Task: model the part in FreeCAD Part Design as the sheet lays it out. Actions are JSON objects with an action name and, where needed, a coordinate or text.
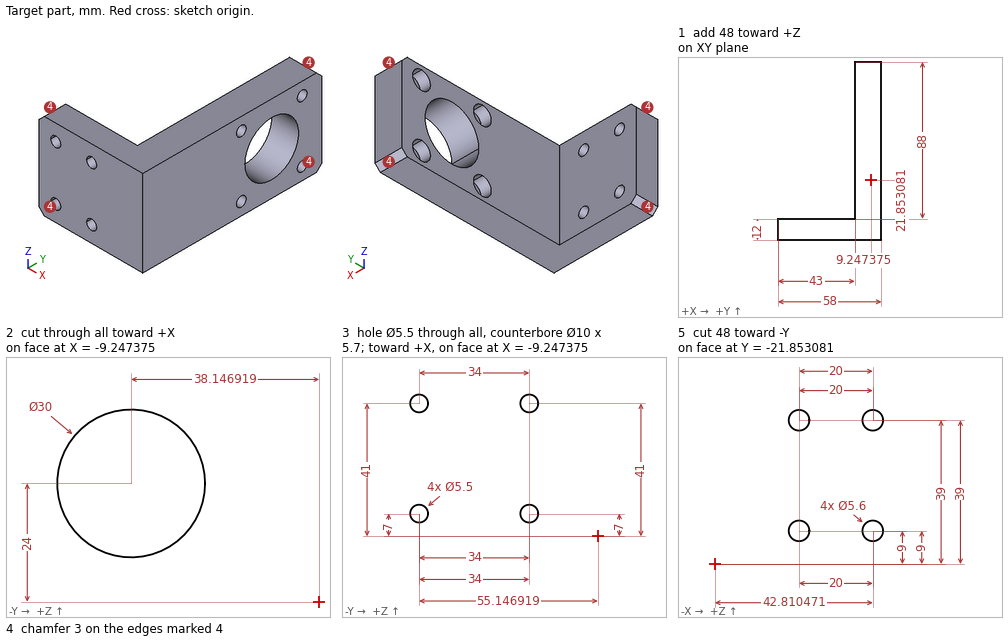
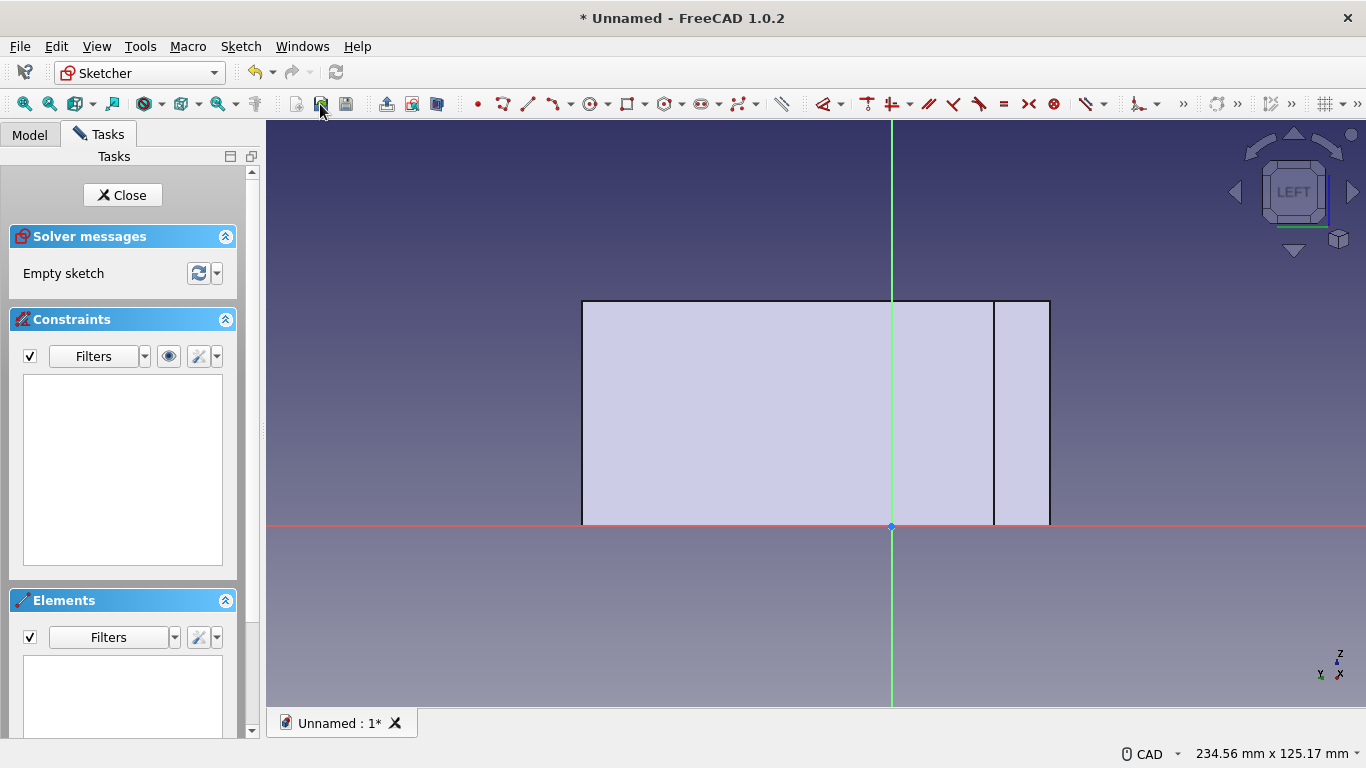
{"action": "scroll", "coordinate": [783, 452], "scroll_direction": "up", "scroll_amount": 4}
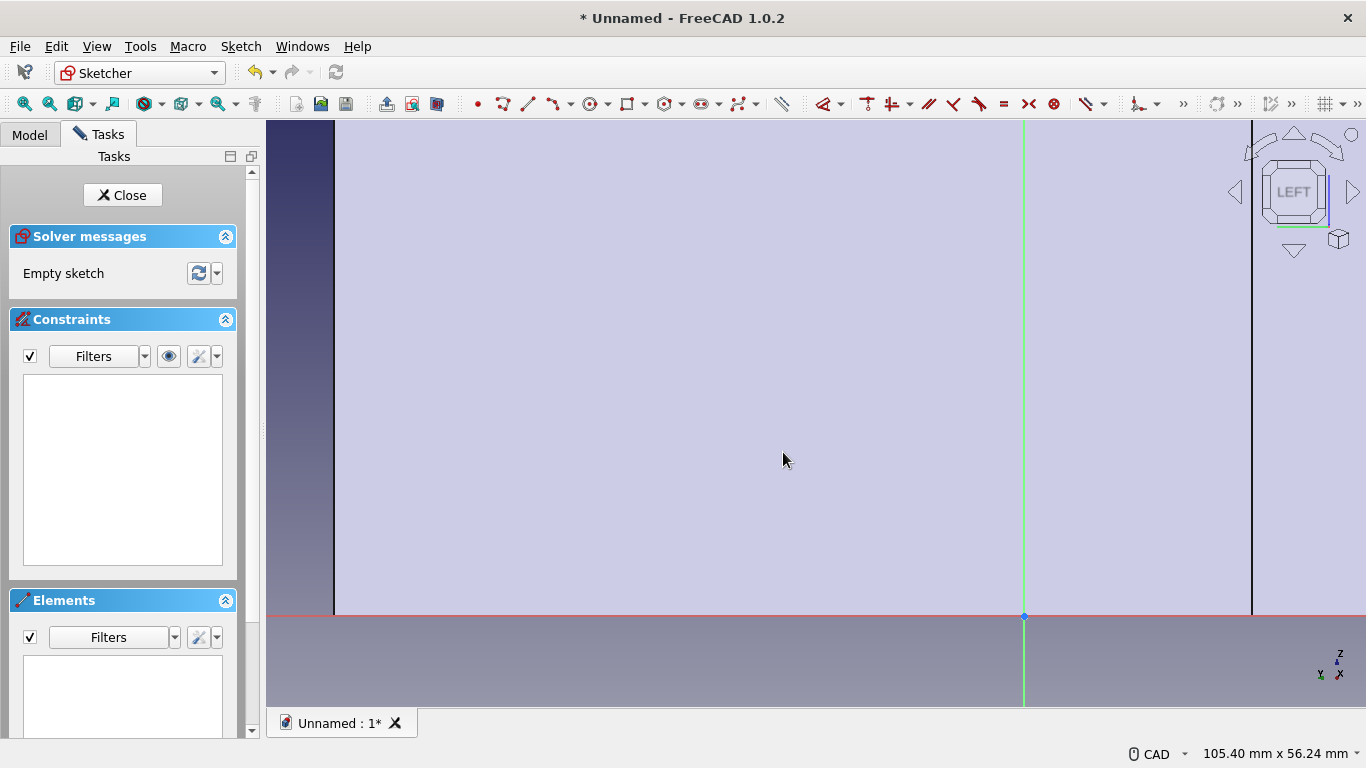
{"action": "left_click", "coordinate": [590, 104]}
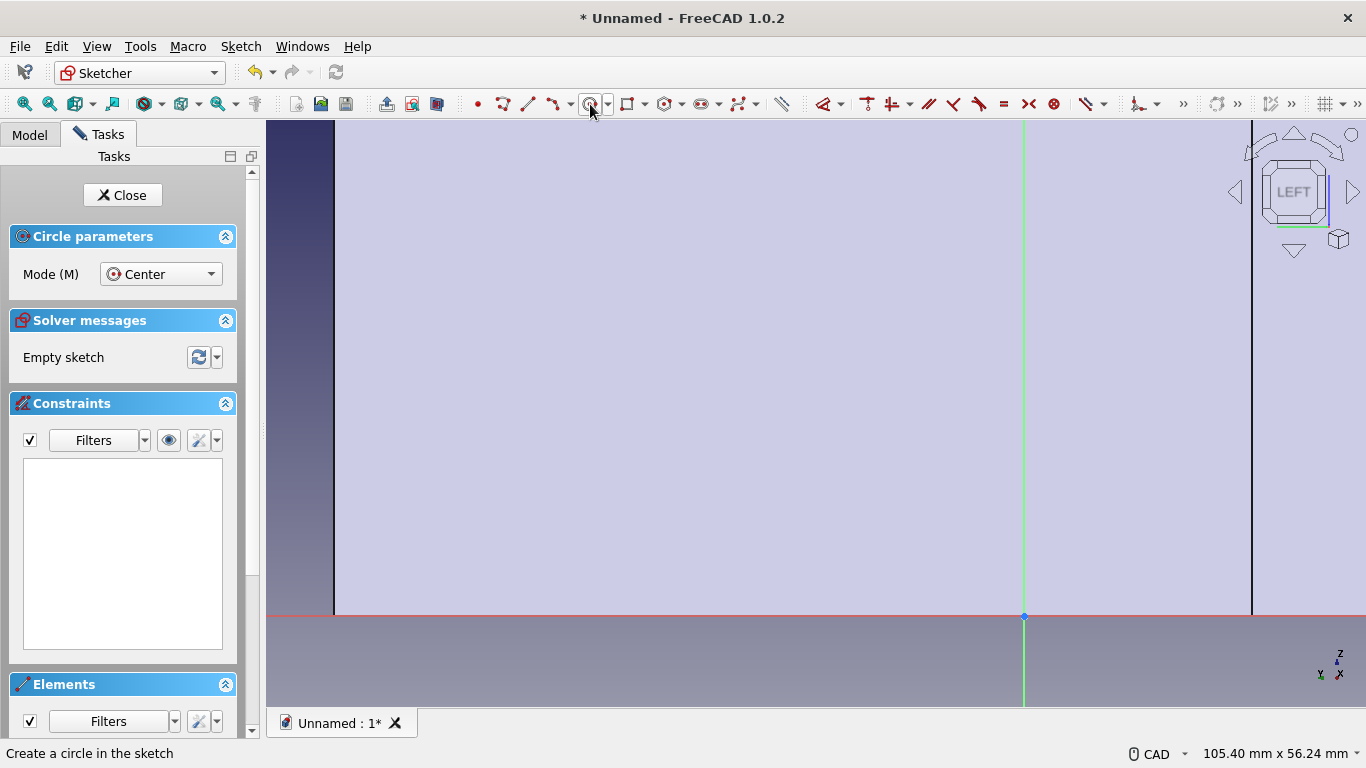
{"action": "left_click", "coordinate": [626, 366]}
{"action": "left_click", "coordinate": [737, 255]}
{"action": "key", "text": "Escape"}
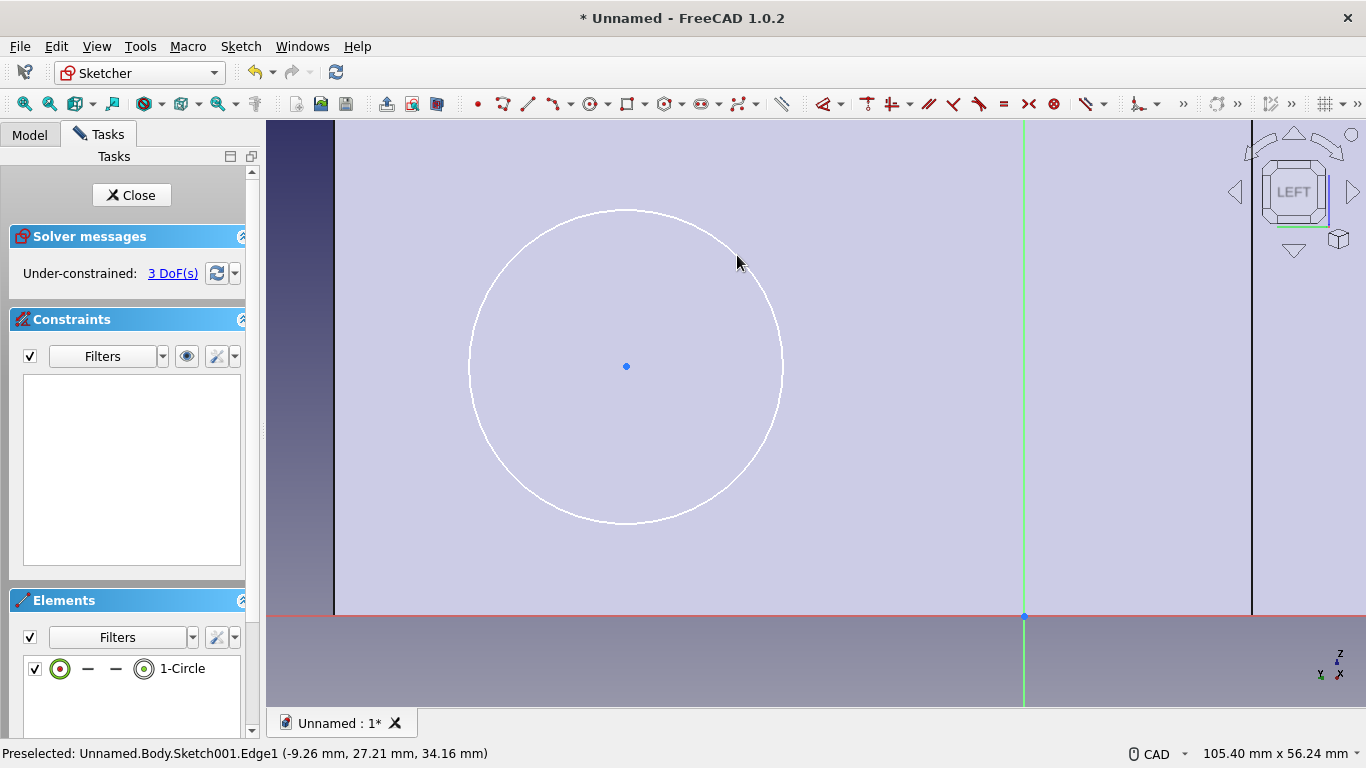
{"action": "left_click", "coordinate": [822, 104]}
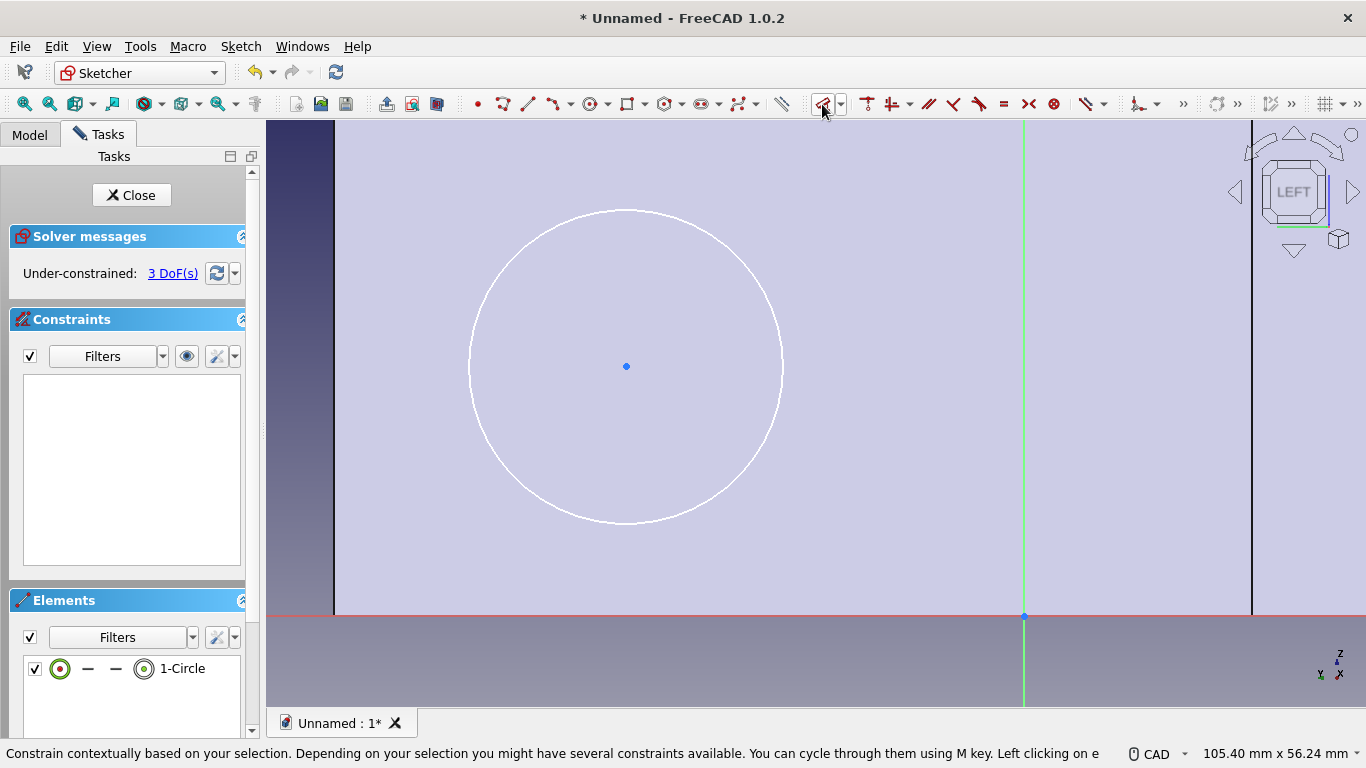
{"action": "left_click", "coordinate": [737, 256]}
{"action": "left_click", "coordinate": [760, 233]}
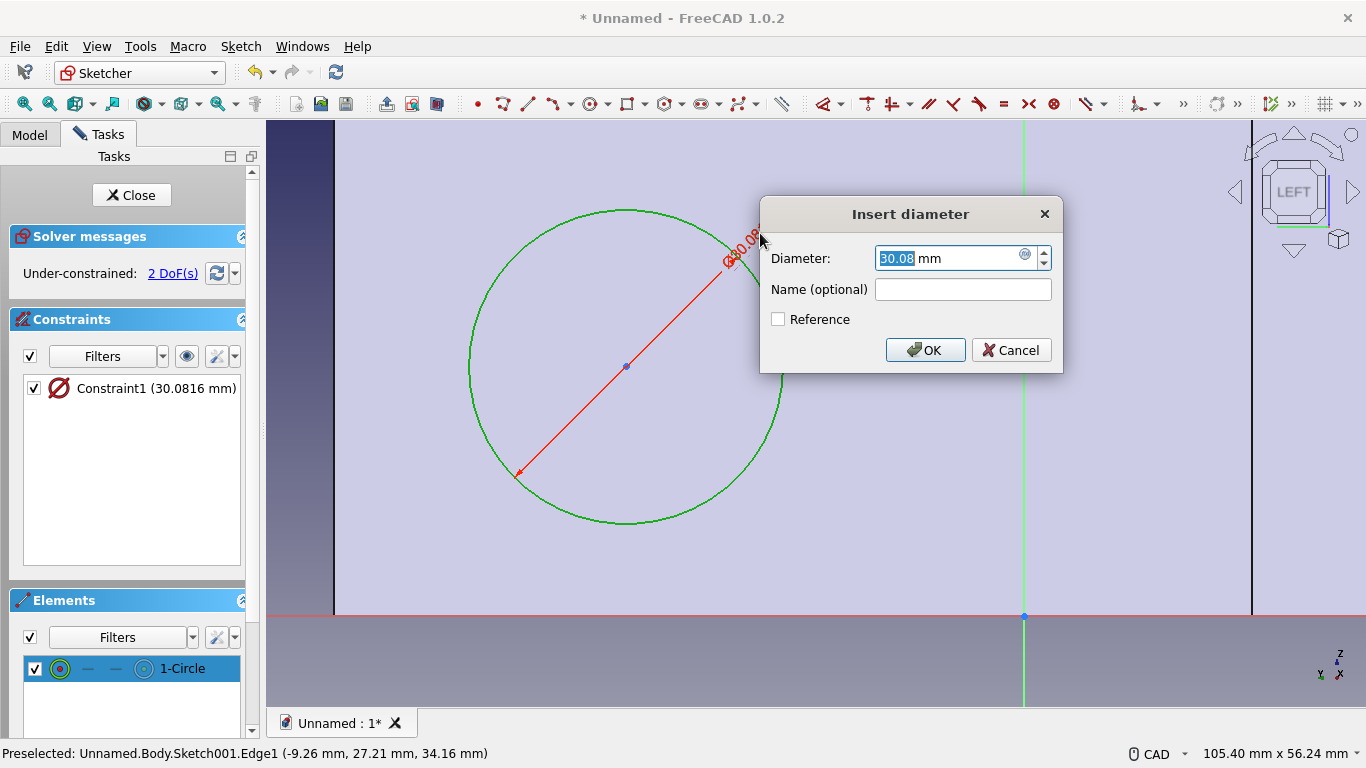
{"action": "type", "text": "30"}
{"action": "key", "text": "Return"}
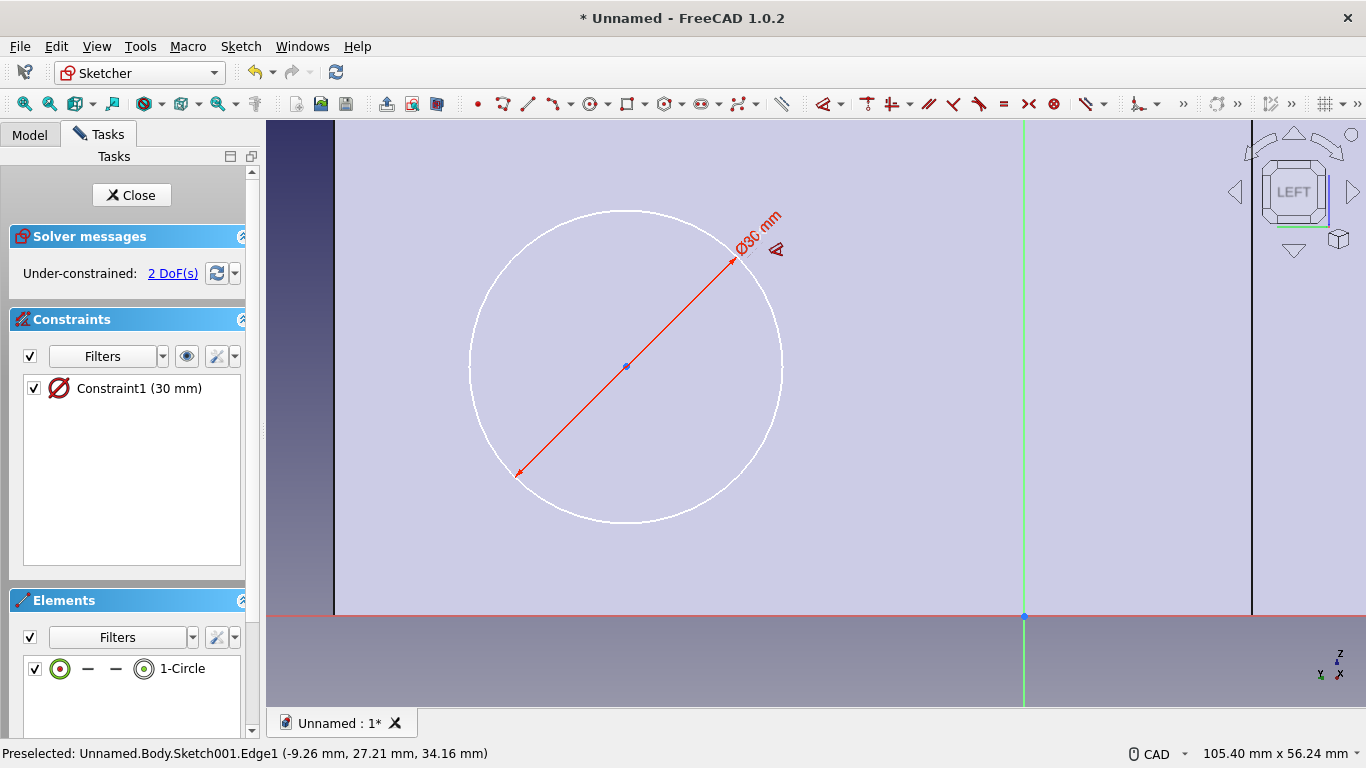
{"action": "left_click", "coordinate": [626, 367]}
{"action": "left_click", "coordinate": [1058, 492]}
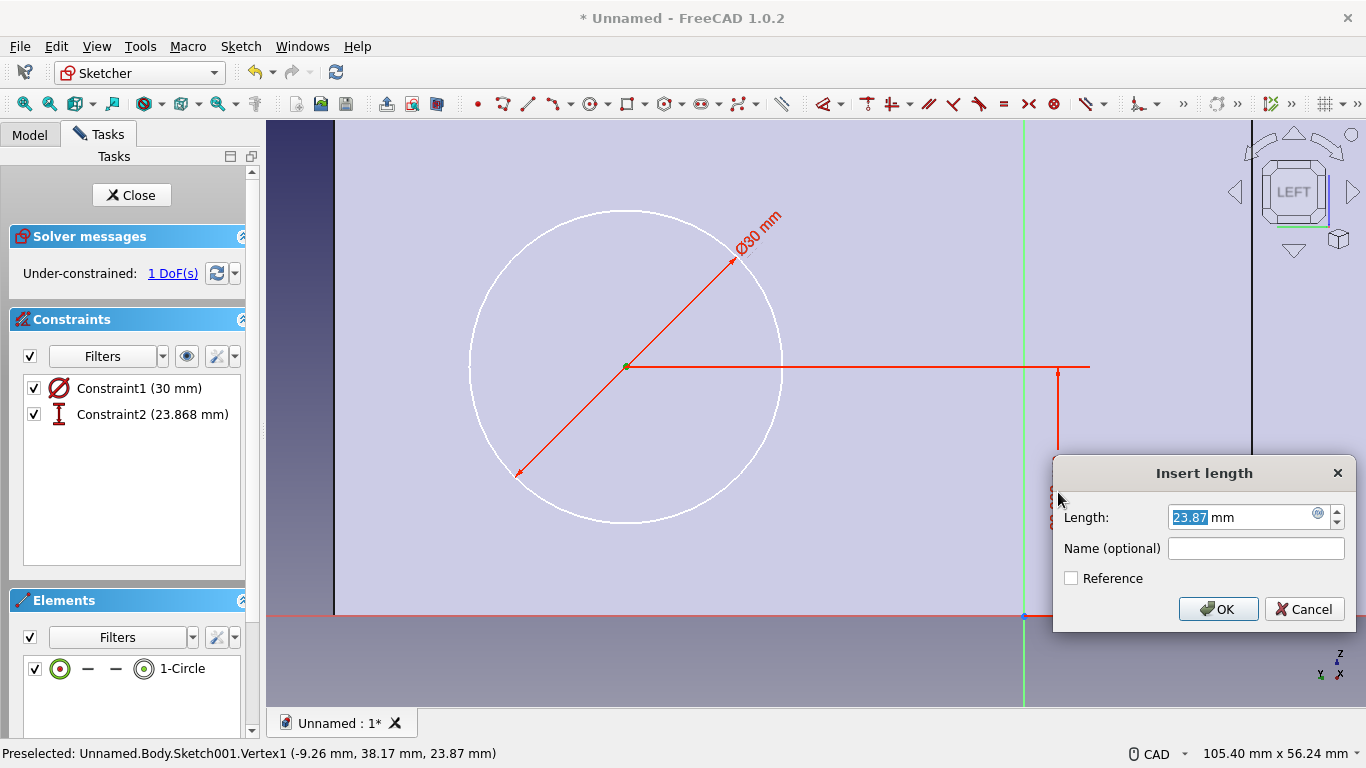
{"action": "type", "text": "24"}
{"action": "key", "text": "Return"}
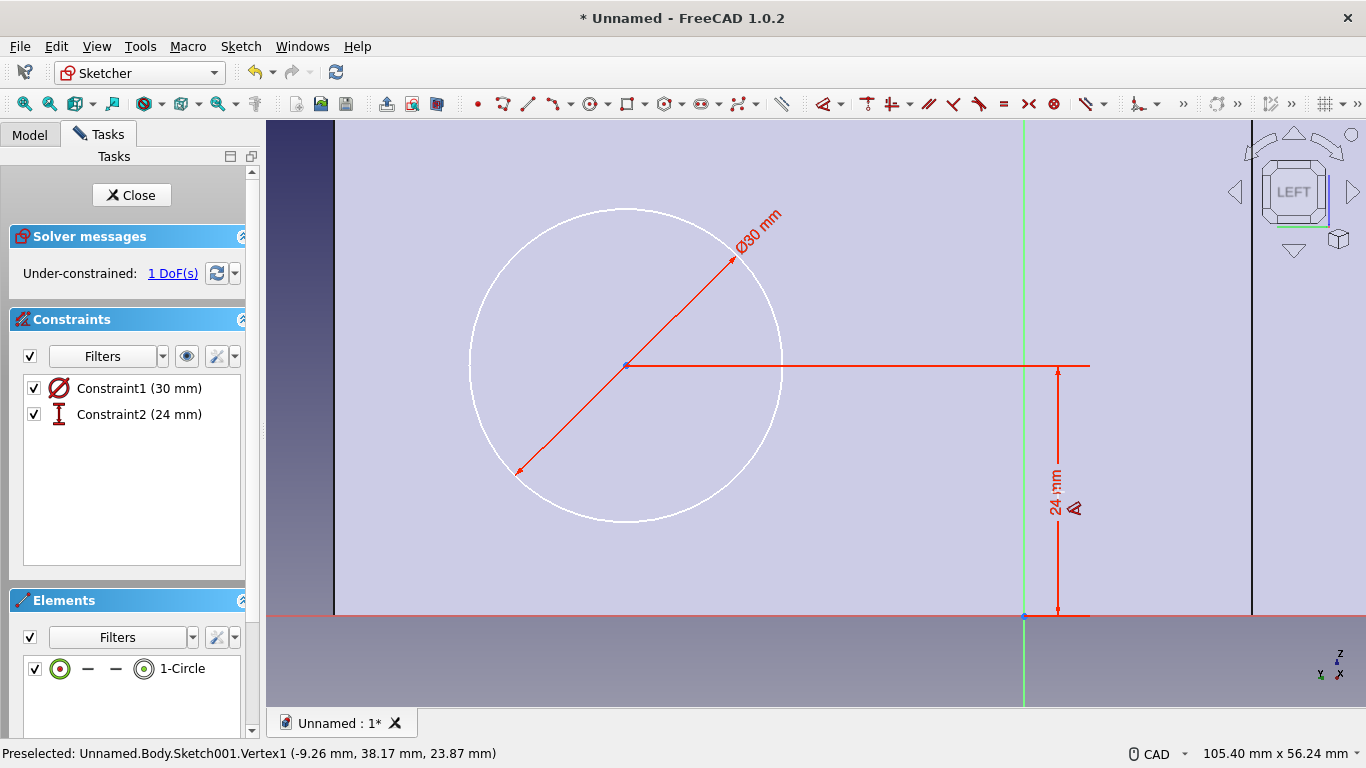
{"action": "left_click", "coordinate": [626, 366]}
{"action": "left_click", "coordinate": [825, 650]}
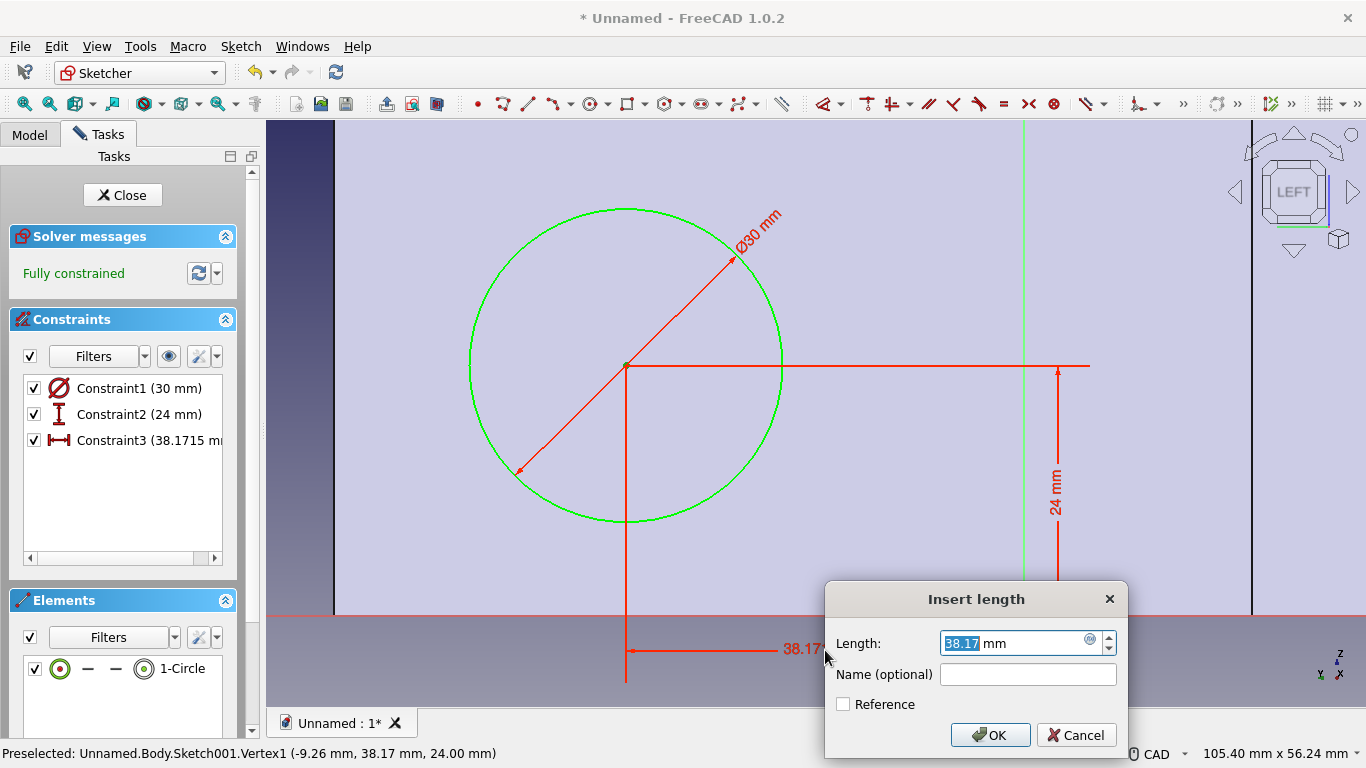
{"action": "type", "text": "38.146919"}
{"action": "key", "text": "Return"}
{"action": "key", "text": "Escape"}